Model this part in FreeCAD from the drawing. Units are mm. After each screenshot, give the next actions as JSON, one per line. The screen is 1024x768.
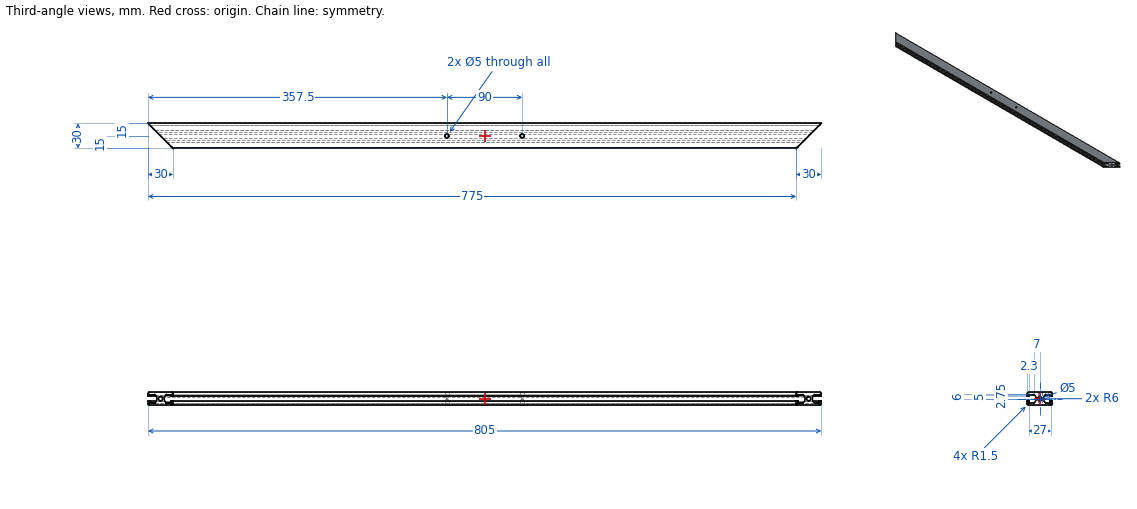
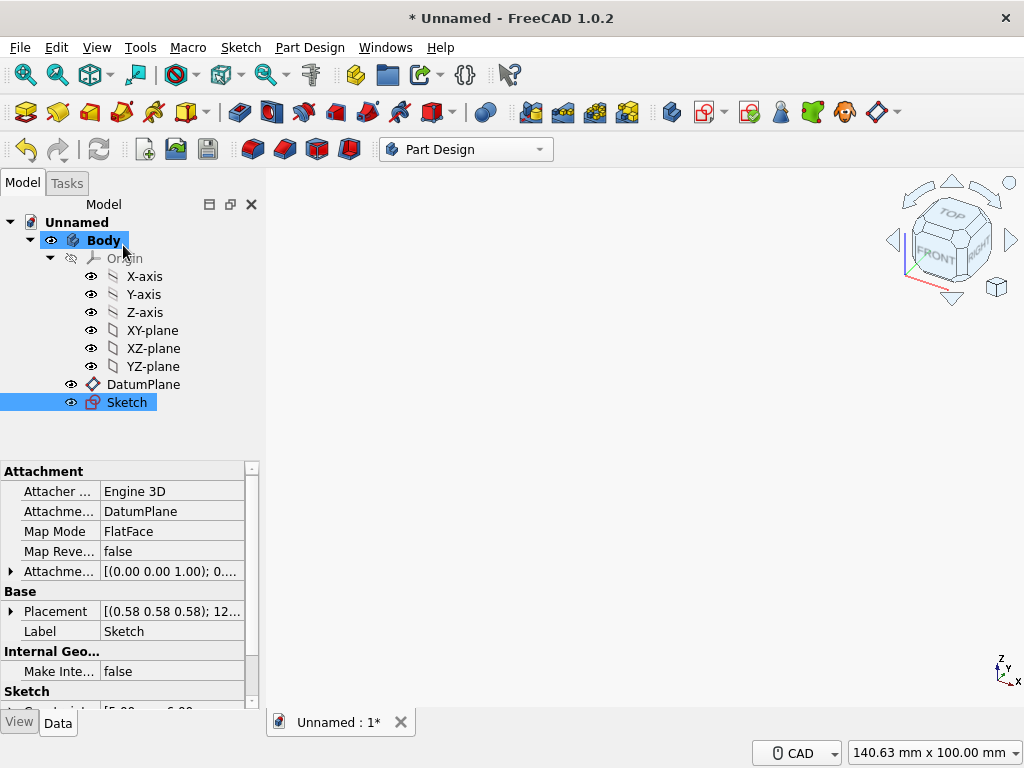
{"action": "left_click", "coordinate": [26, 112]}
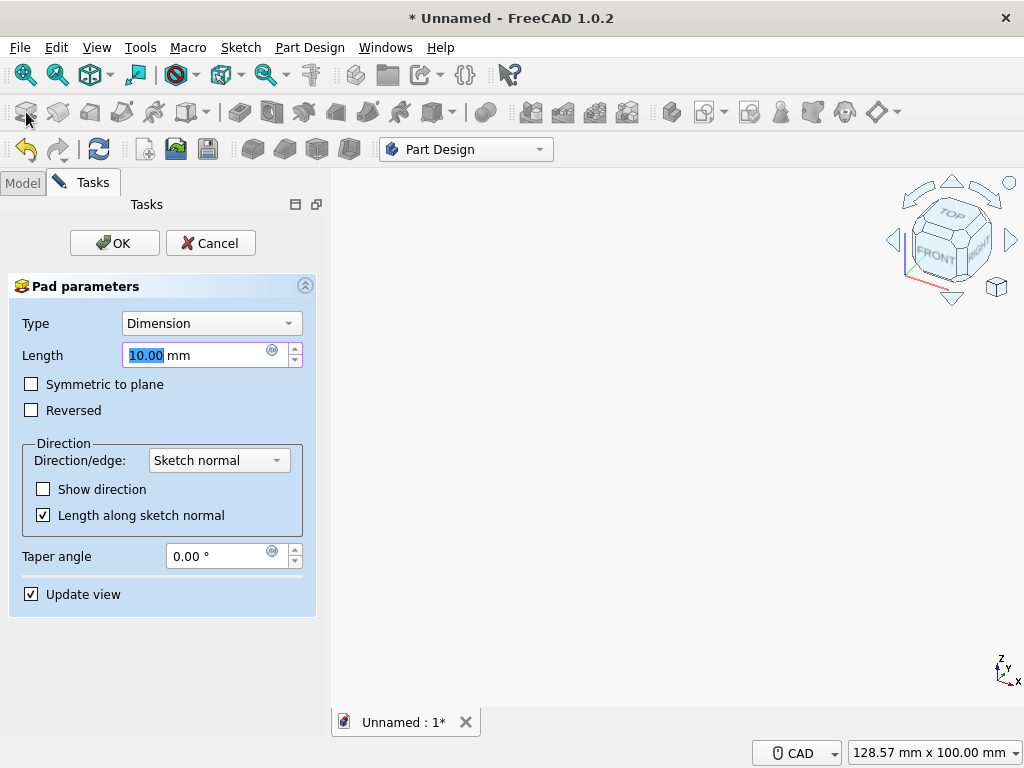
{"action": "type", "text": "805"}
{"action": "key", "text": "Tab"}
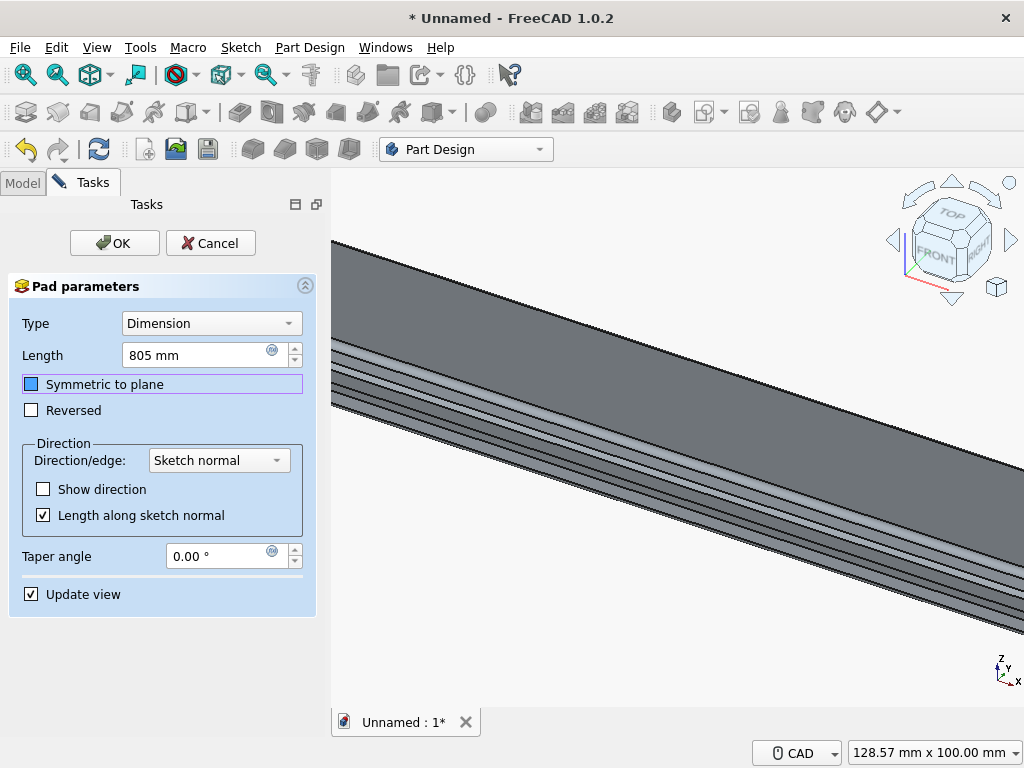
{"action": "left_click", "coordinate": [115, 243]}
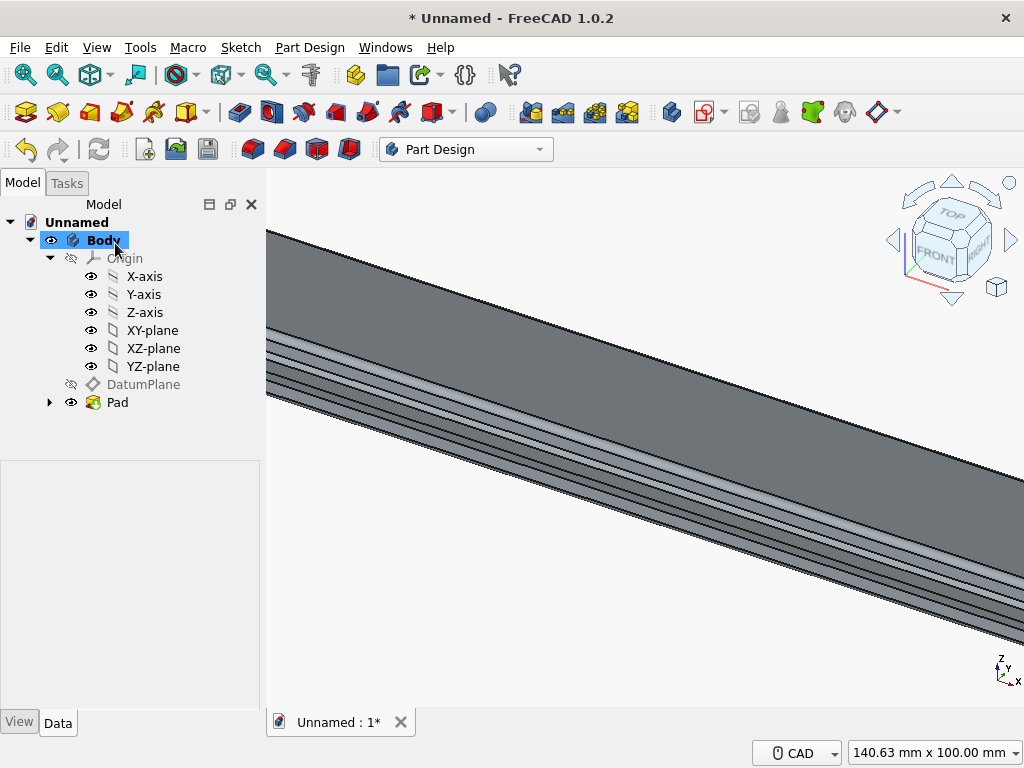
{"action": "left_click", "coordinate": [26, 76]}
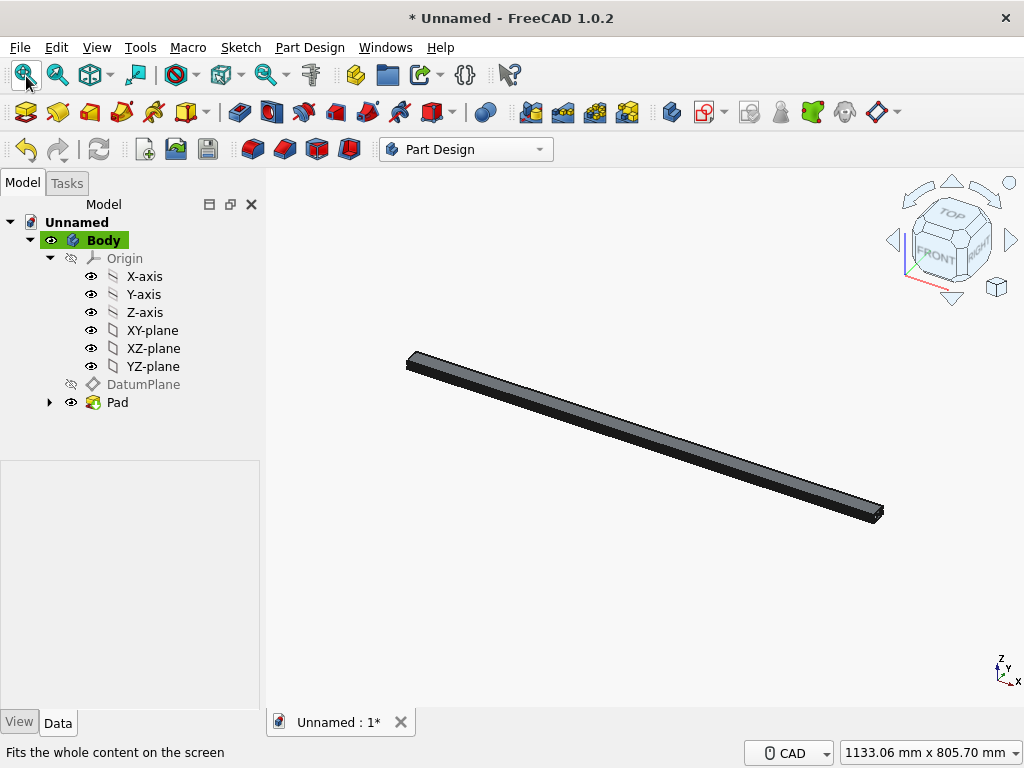
{"action": "key", "text": "0"}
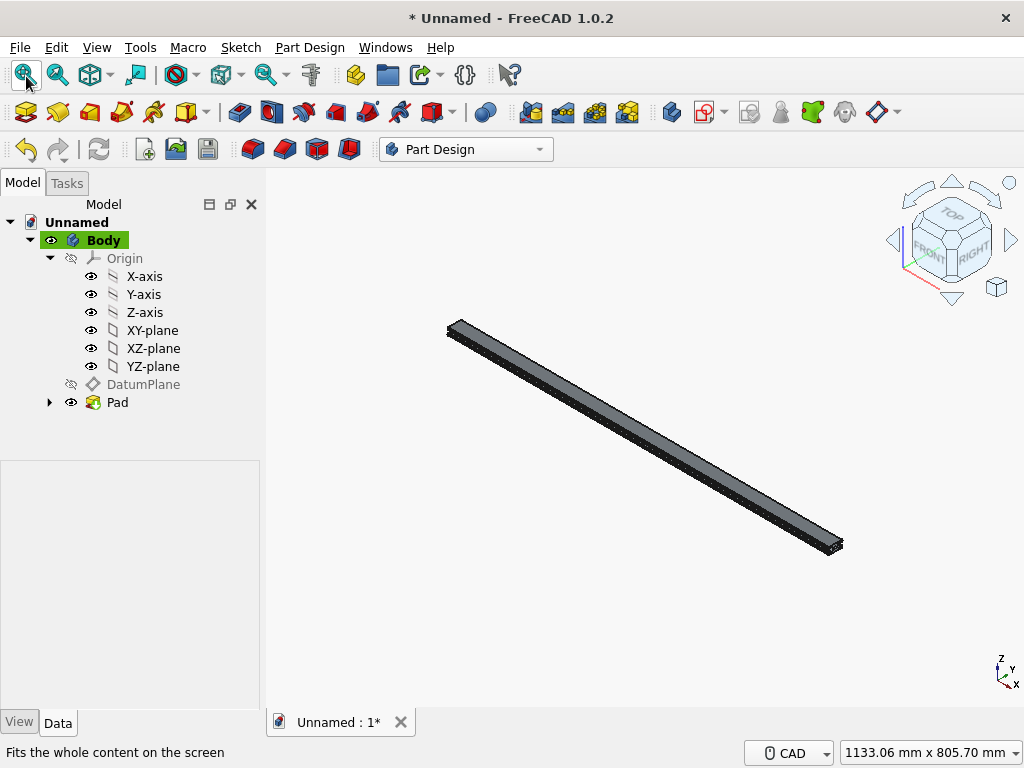
{"action": "key", "text": "2"}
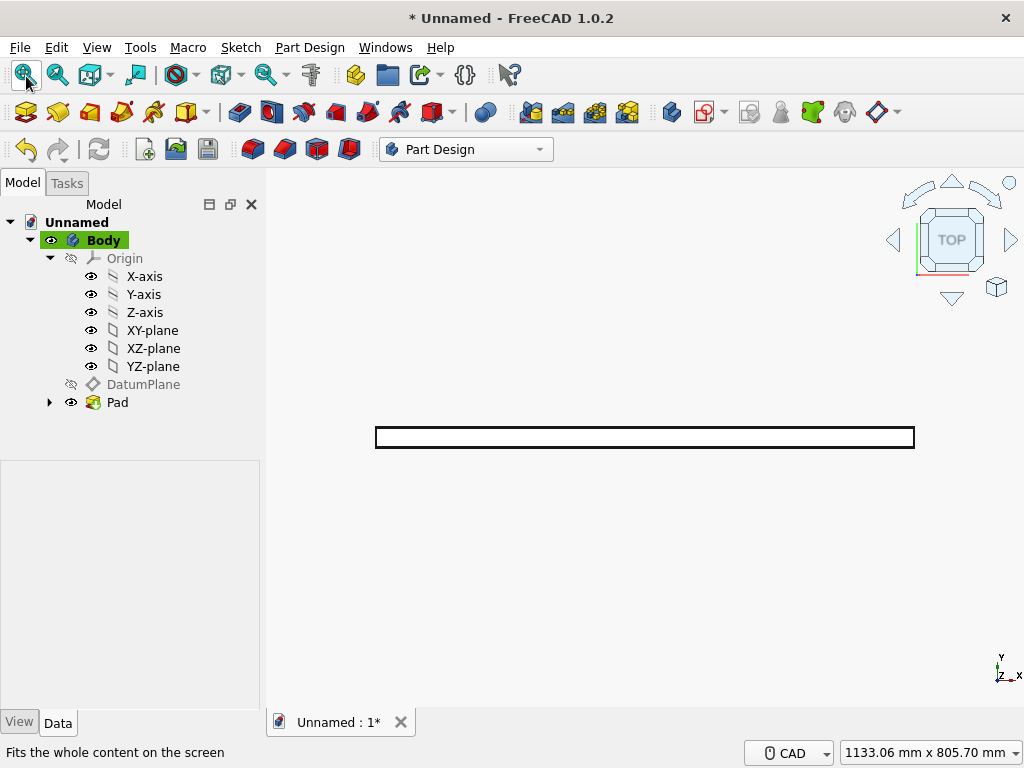
{"action": "left_click", "coordinate": [645, 436]}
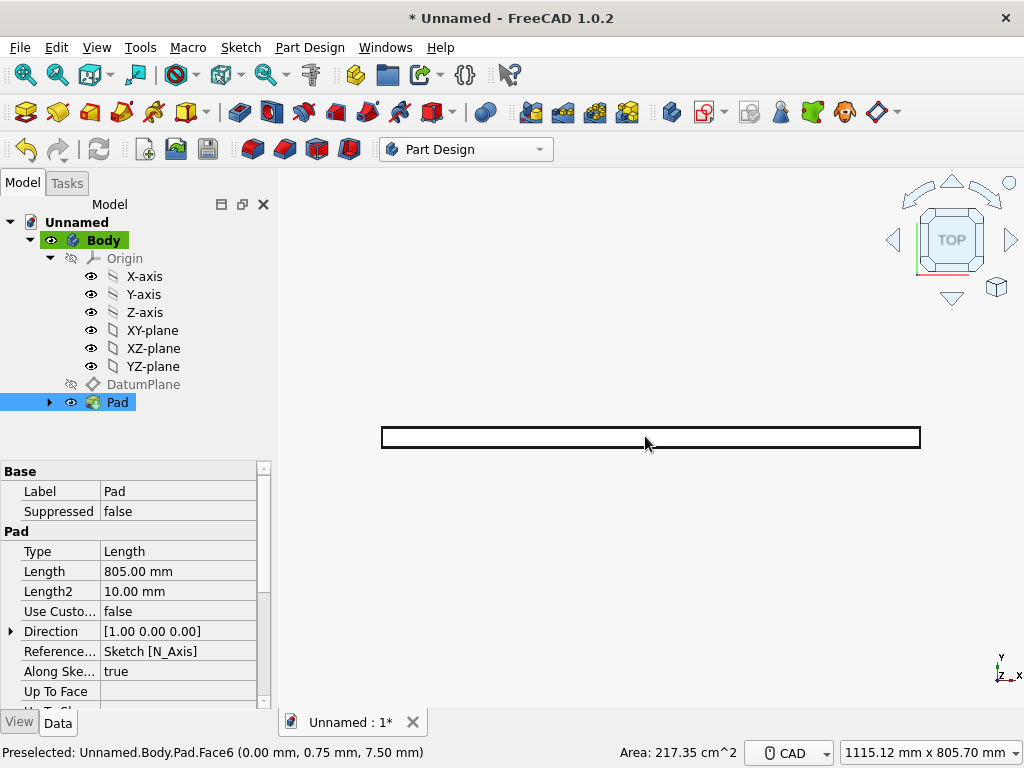
{"action": "left_click", "coordinate": [704, 112]}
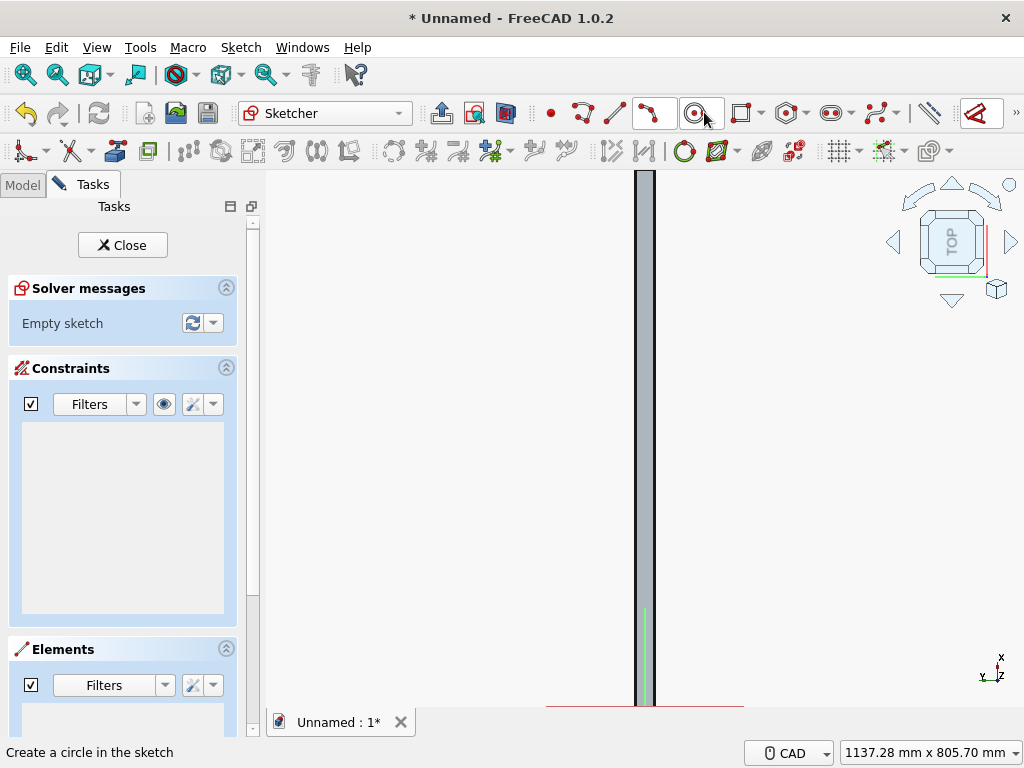
{"action": "scroll", "coordinate": [437, 438], "scroll_direction": "down", "scroll_amount": 2}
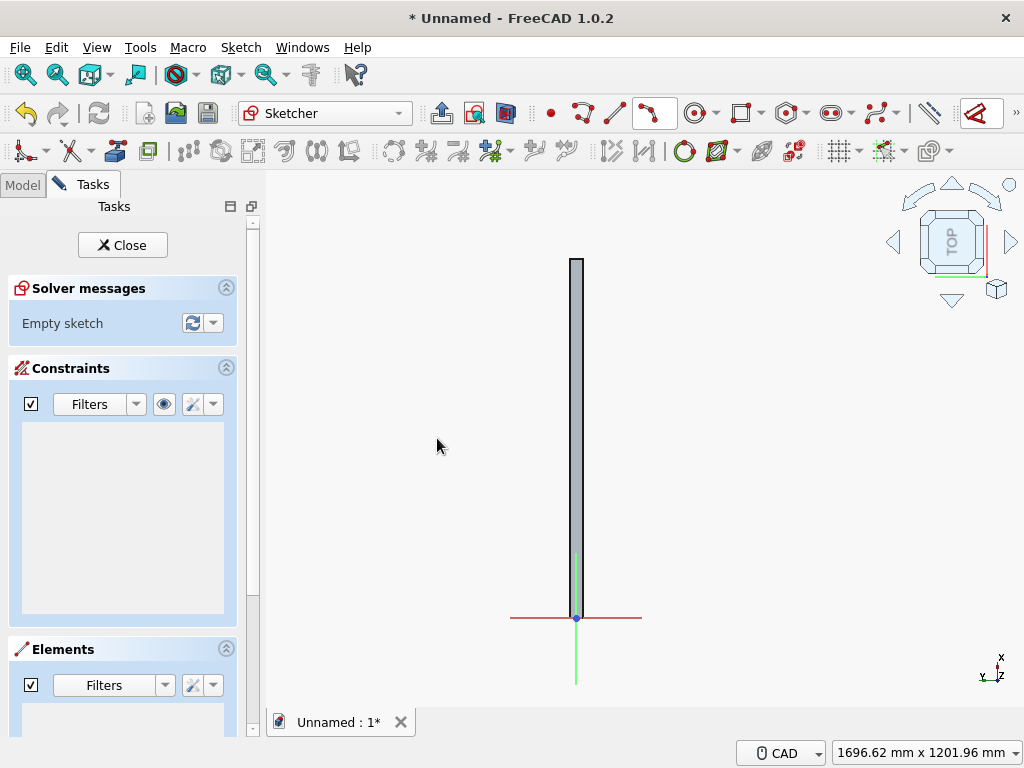
{"action": "left_click", "coordinate": [584, 114]}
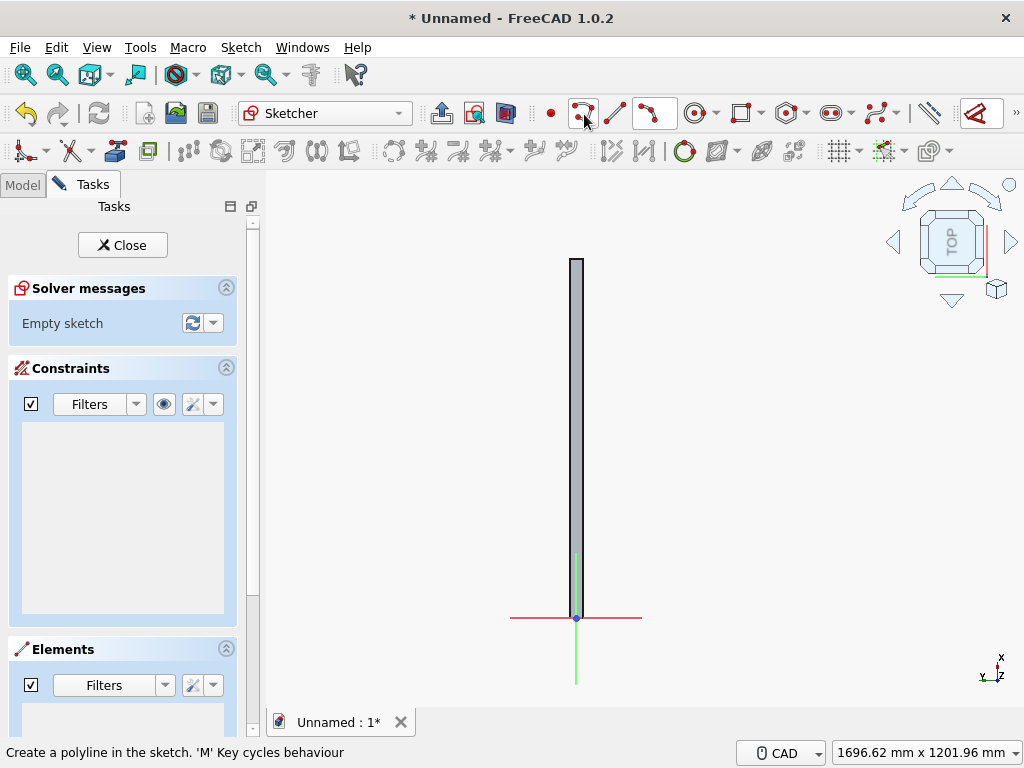
{"action": "scroll", "coordinate": [570, 618], "scroll_direction": "up", "scroll_amount": 5}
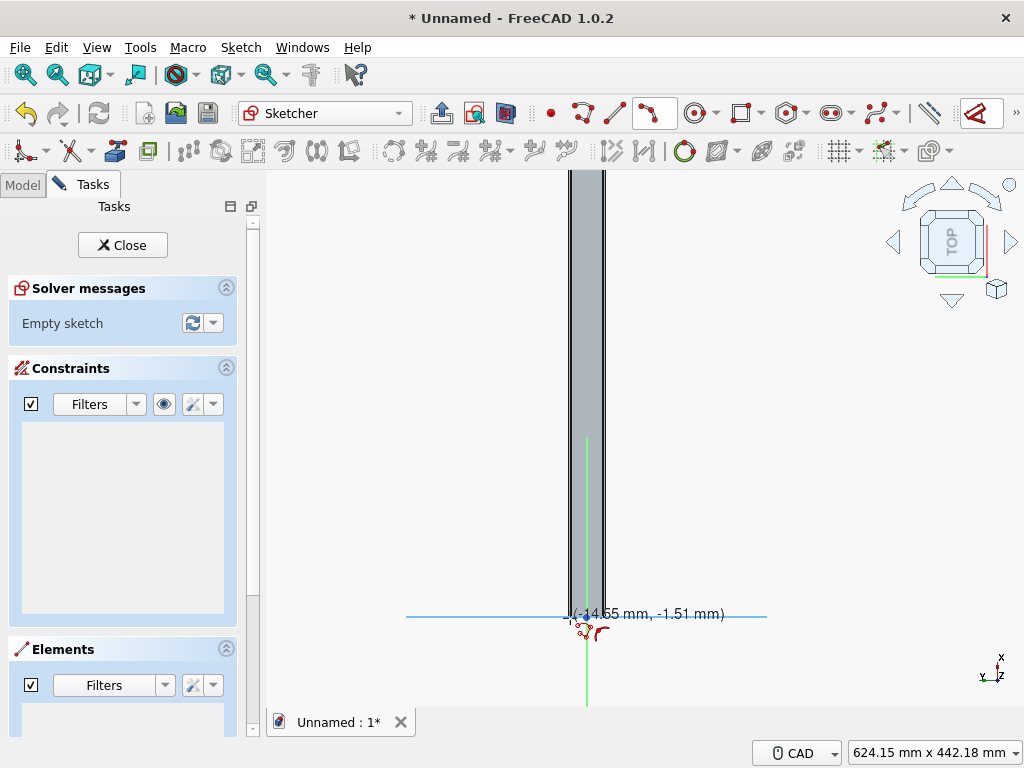
{"action": "left_click", "coordinate": [569, 617]}
{"action": "left_click", "coordinate": [605, 608]}
{"action": "left_click", "coordinate": [605, 581]}
{"action": "left_click", "coordinate": [569, 617]}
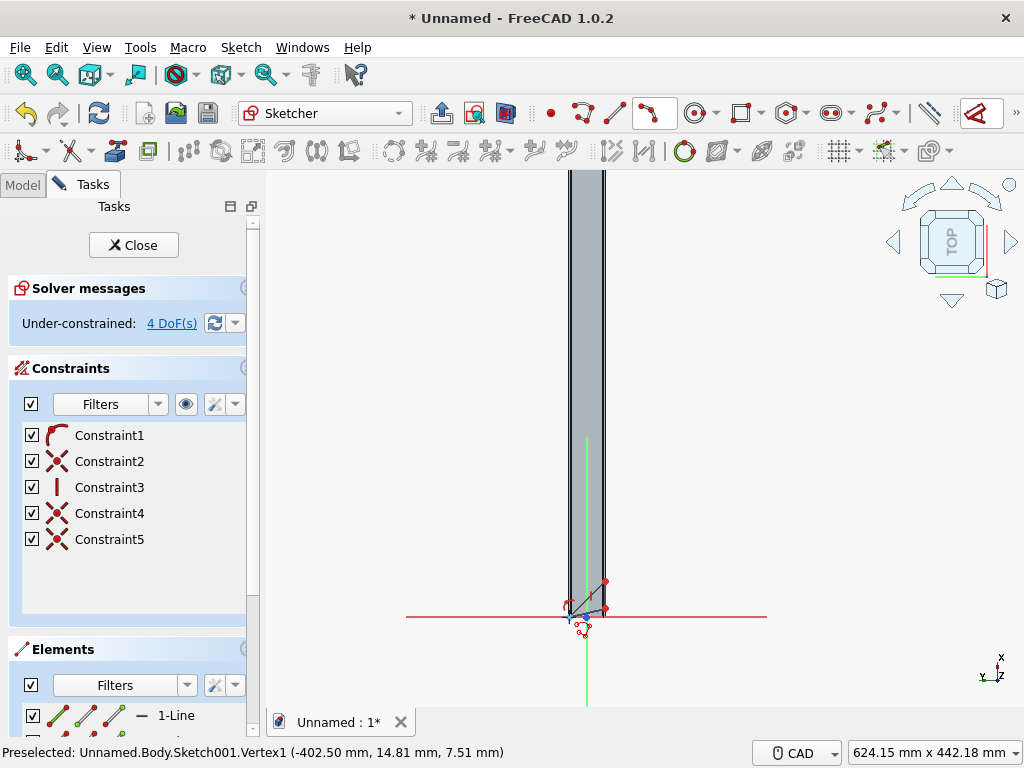
{"action": "scroll", "coordinate": [570, 619], "scroll_direction": "down", "scroll_amount": 5}